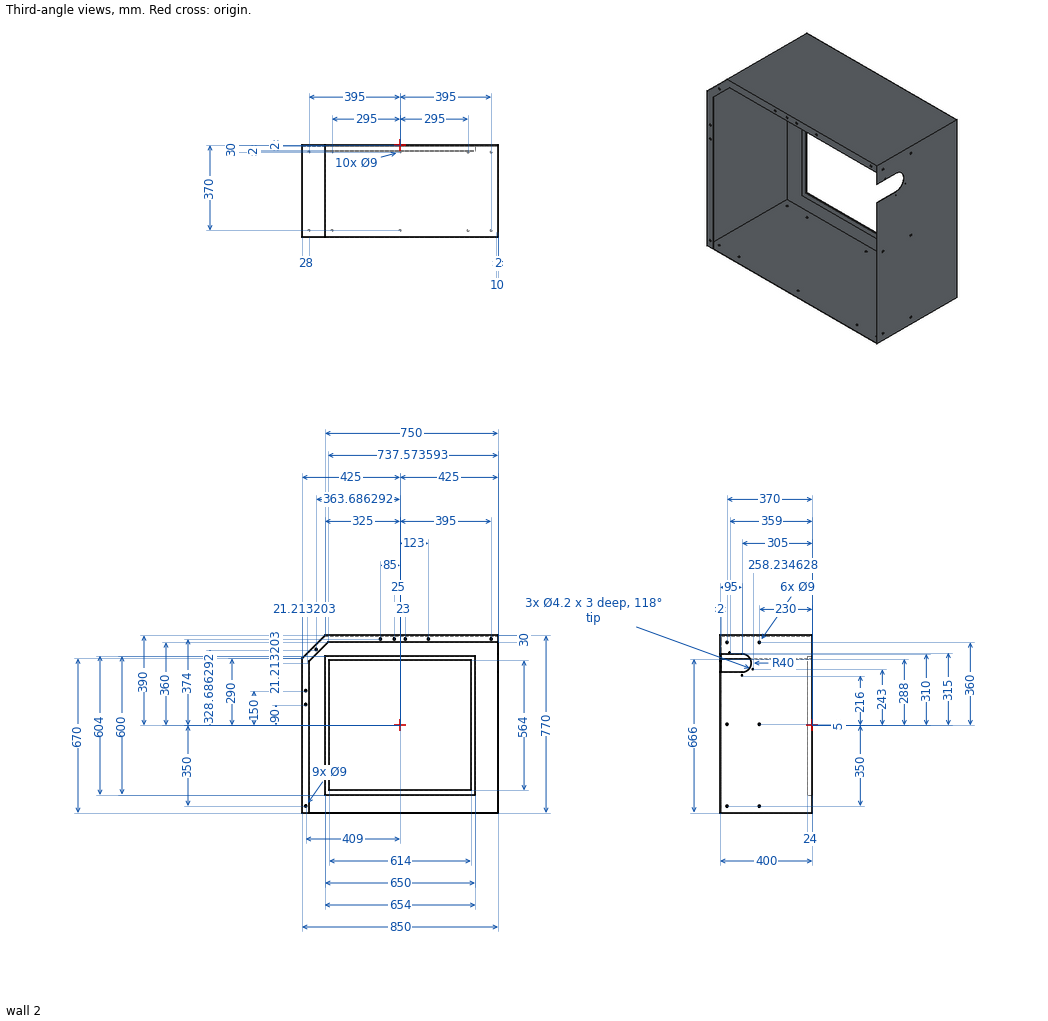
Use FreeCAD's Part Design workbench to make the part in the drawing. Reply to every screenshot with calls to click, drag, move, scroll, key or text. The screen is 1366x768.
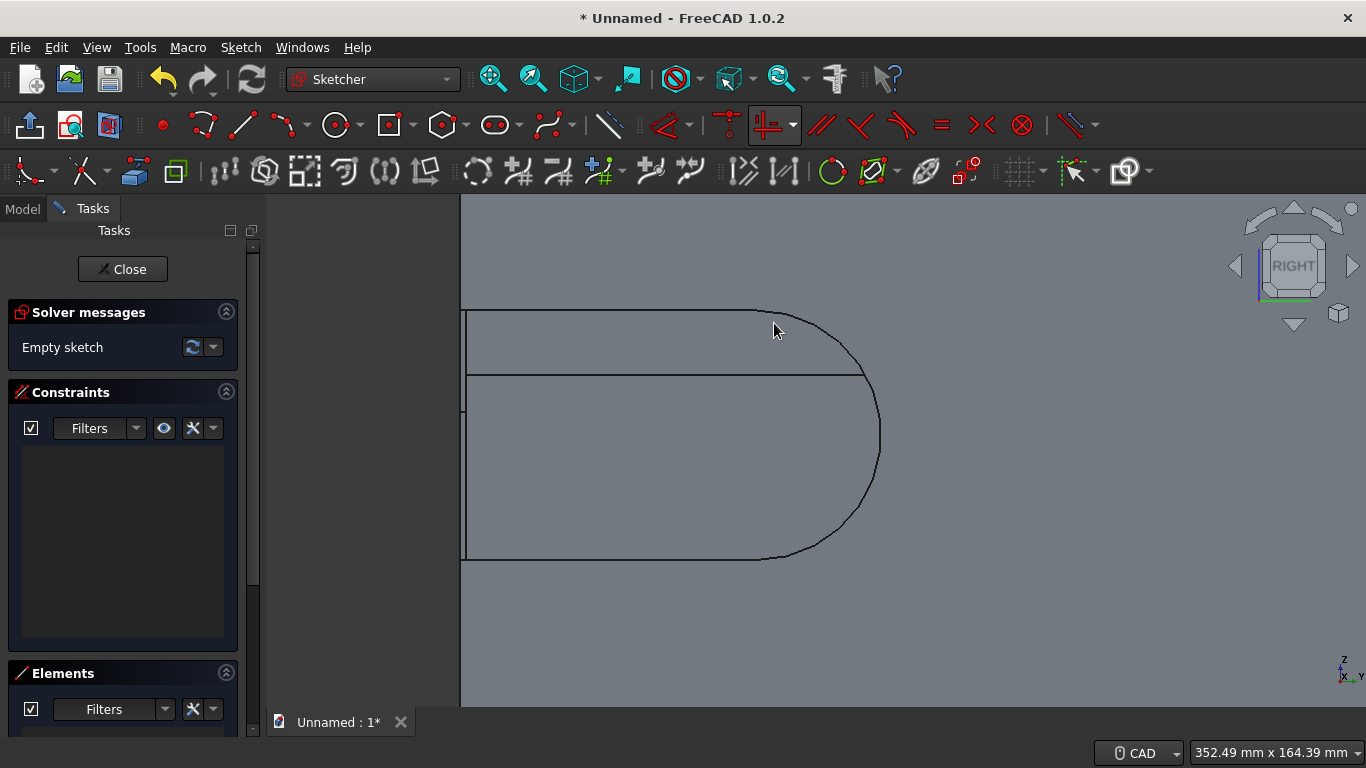
click(336, 126)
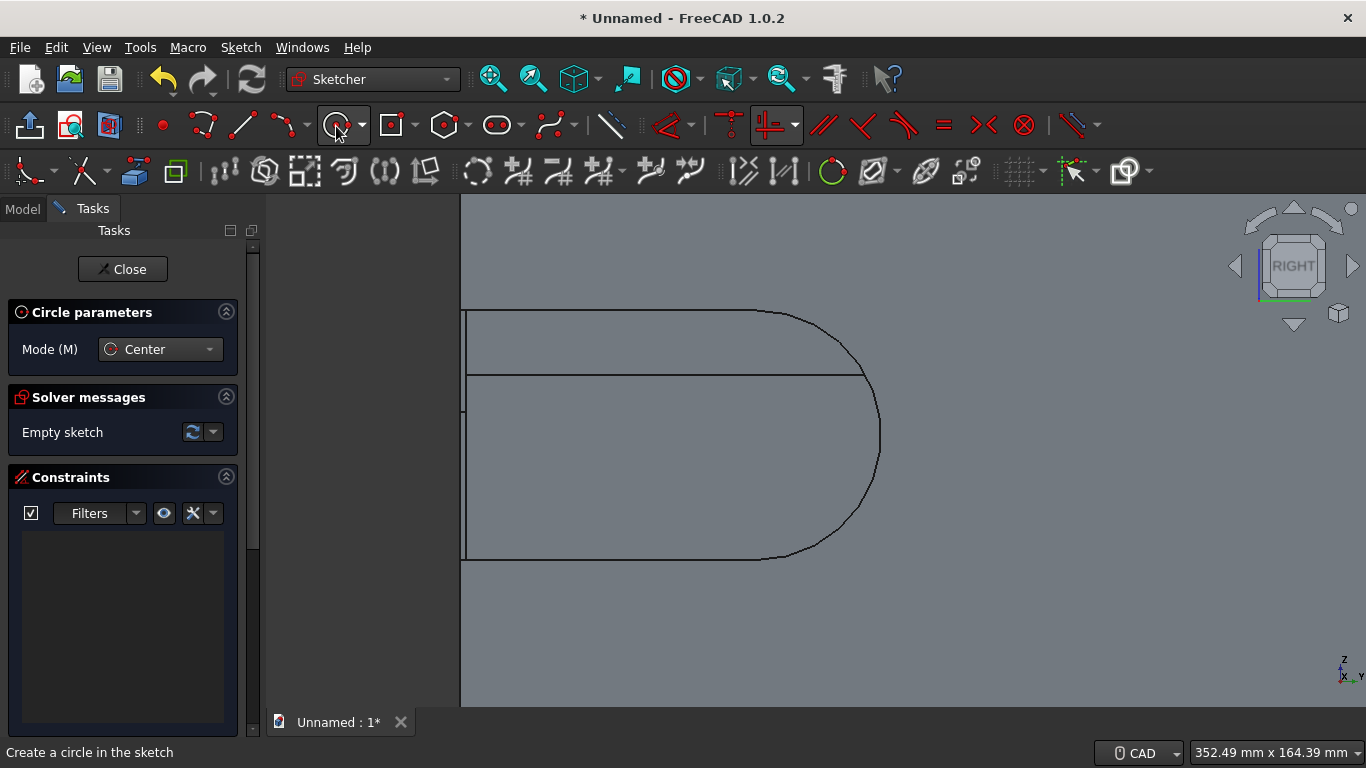
scroll(902, 520, up, 7)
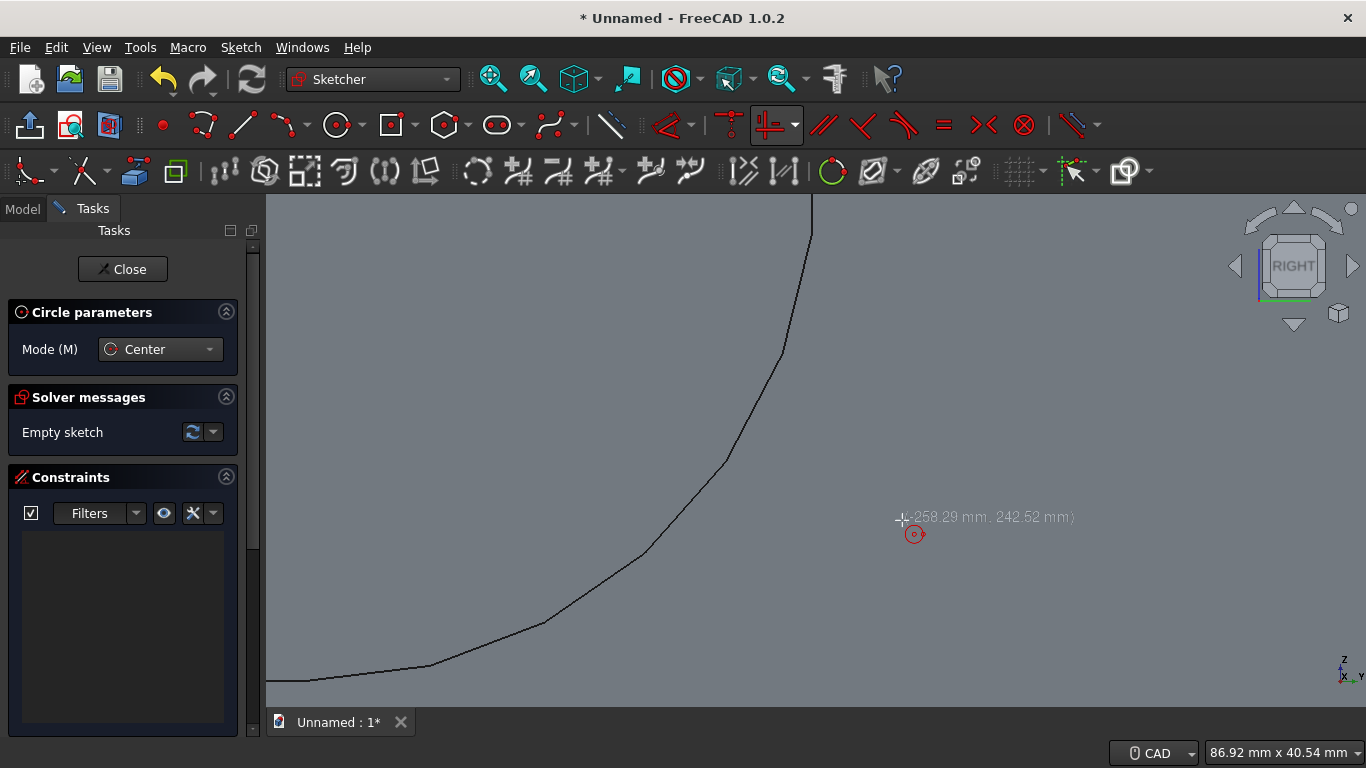
scroll(906, 522, down, 7)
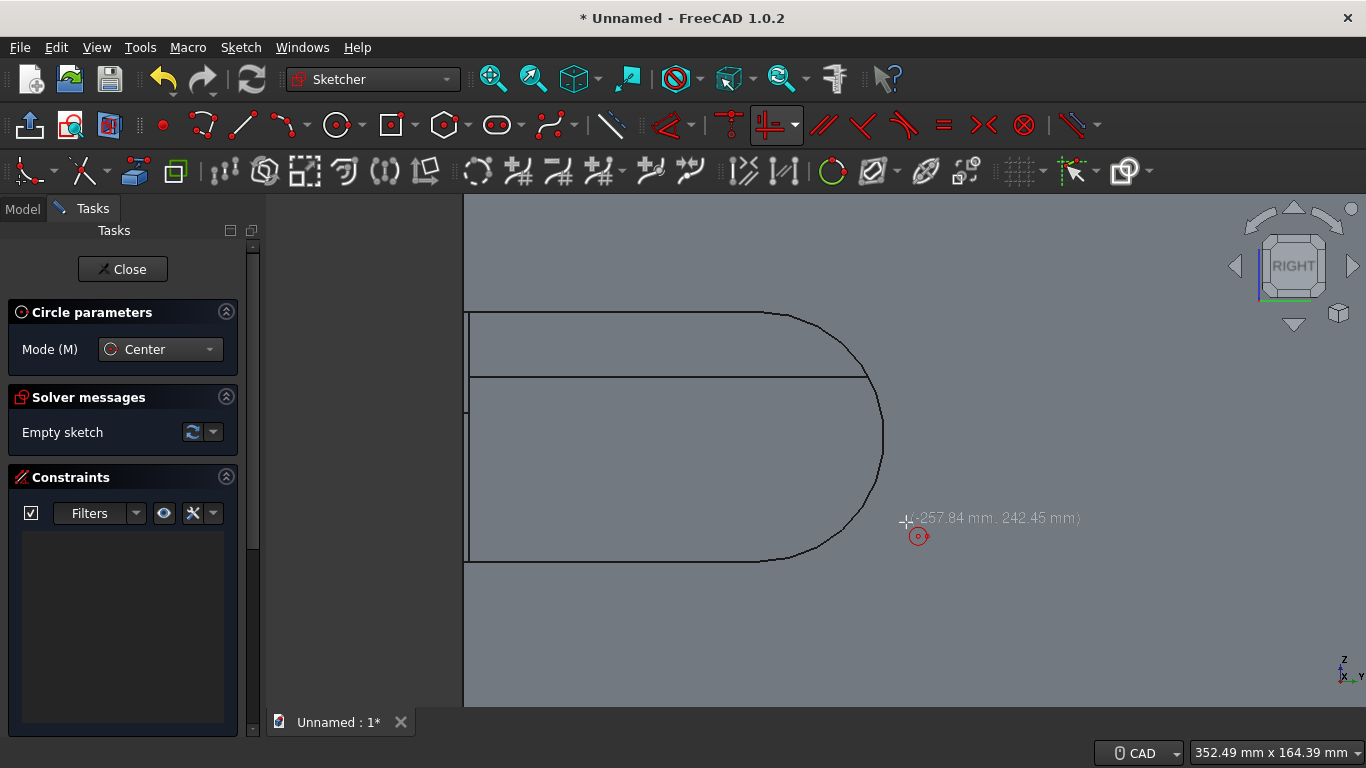
click(905, 521)
move(910, 516)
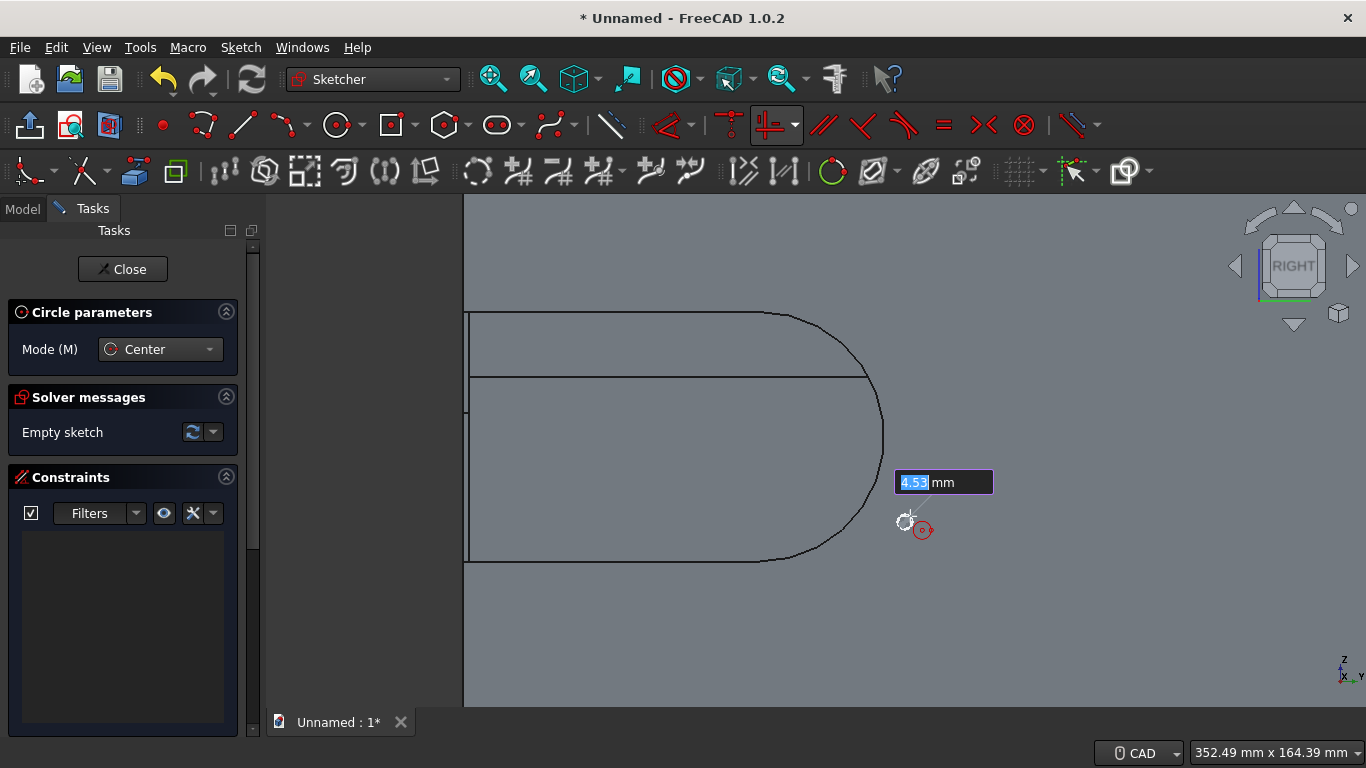
text(4.2)
key(Return)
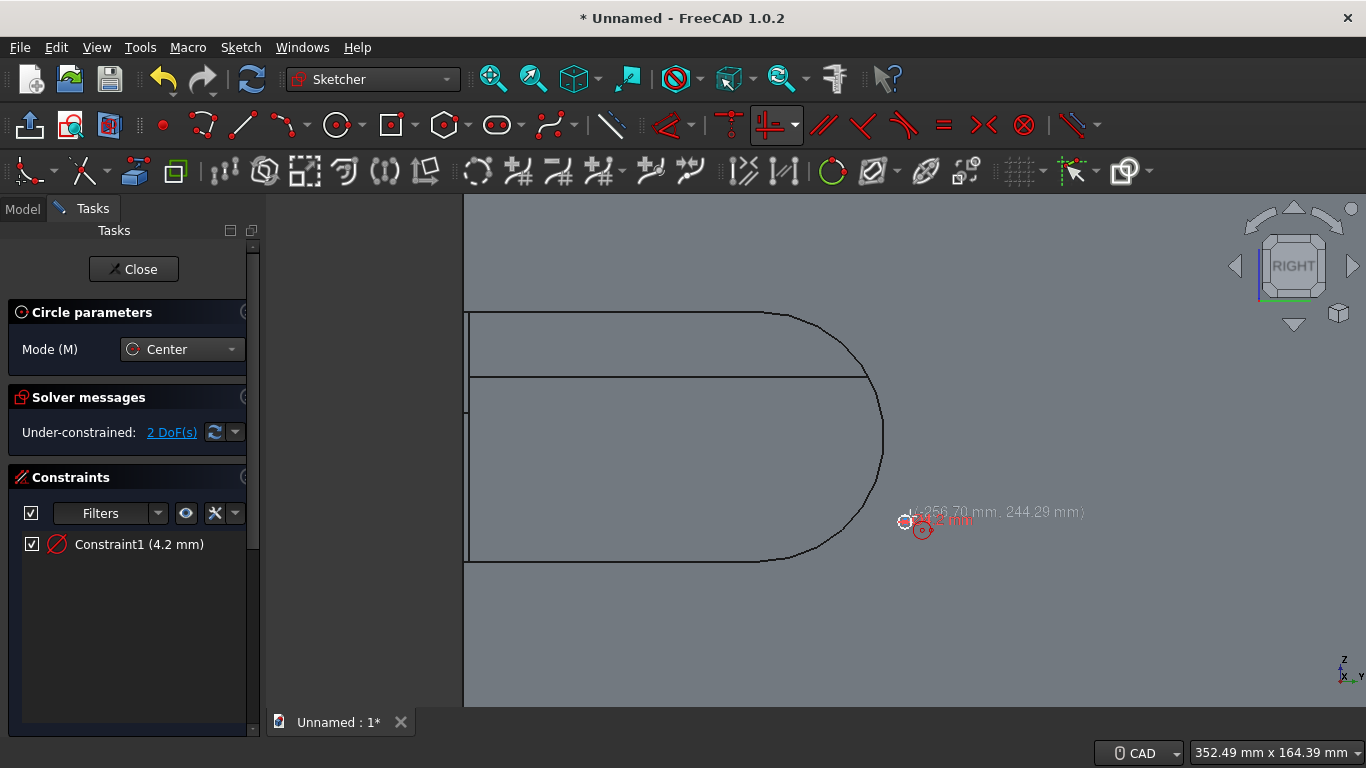
scroll(759, 605, up, 7)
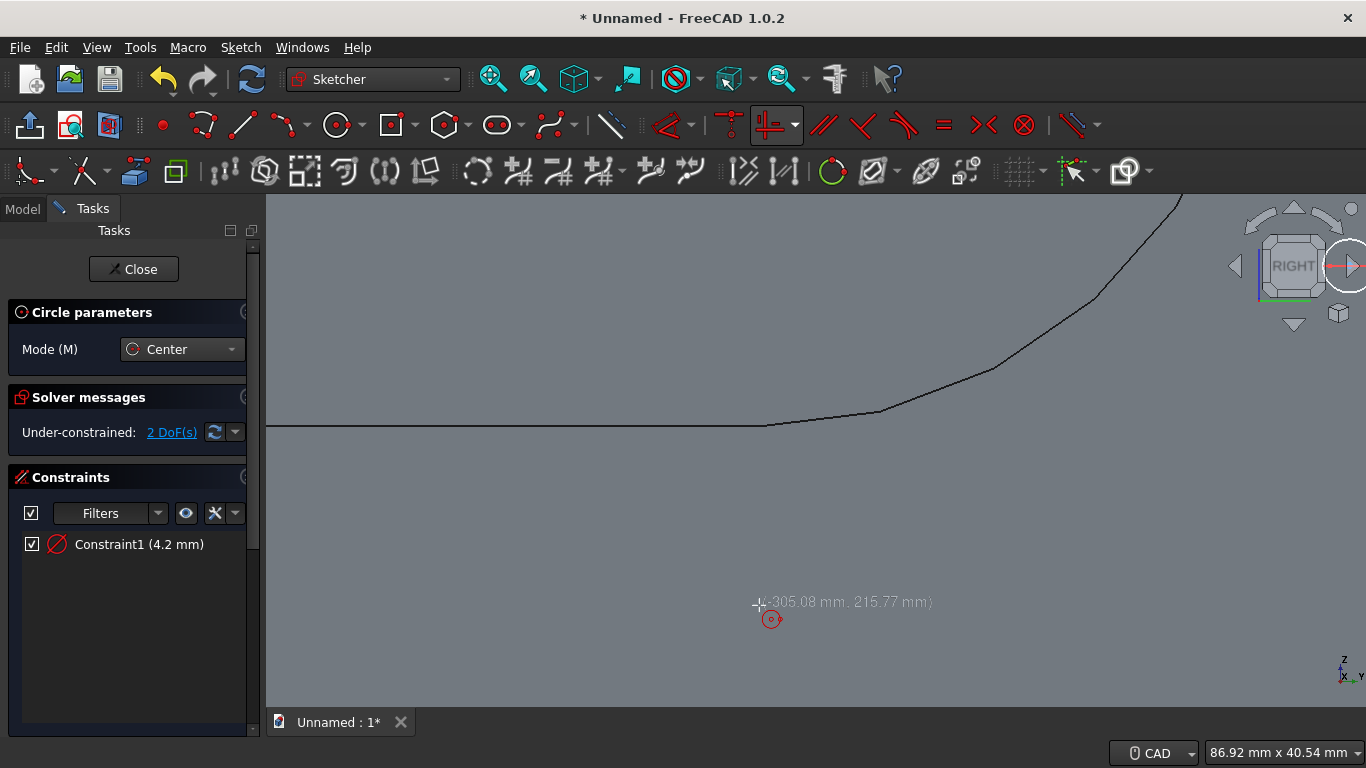
scroll(759, 605, down, 7)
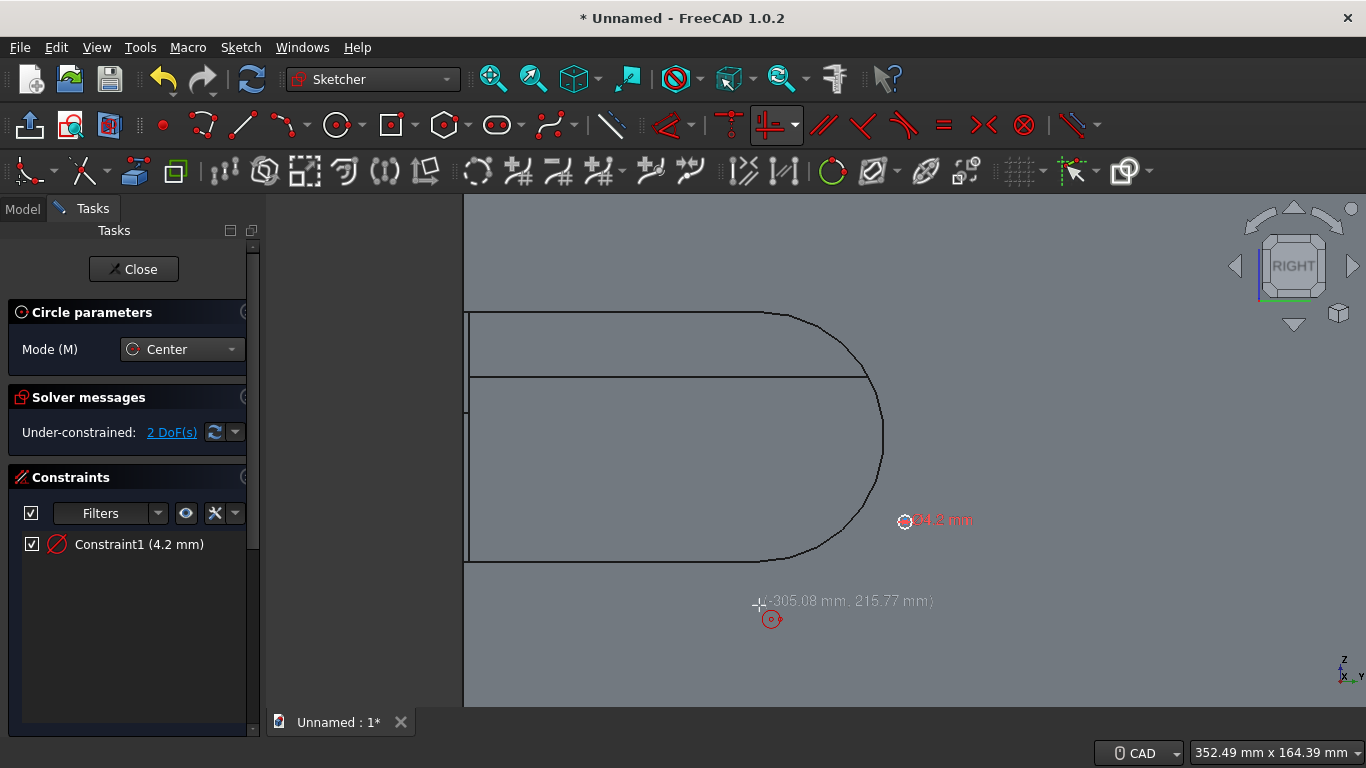
click(759, 605)
move(764, 601)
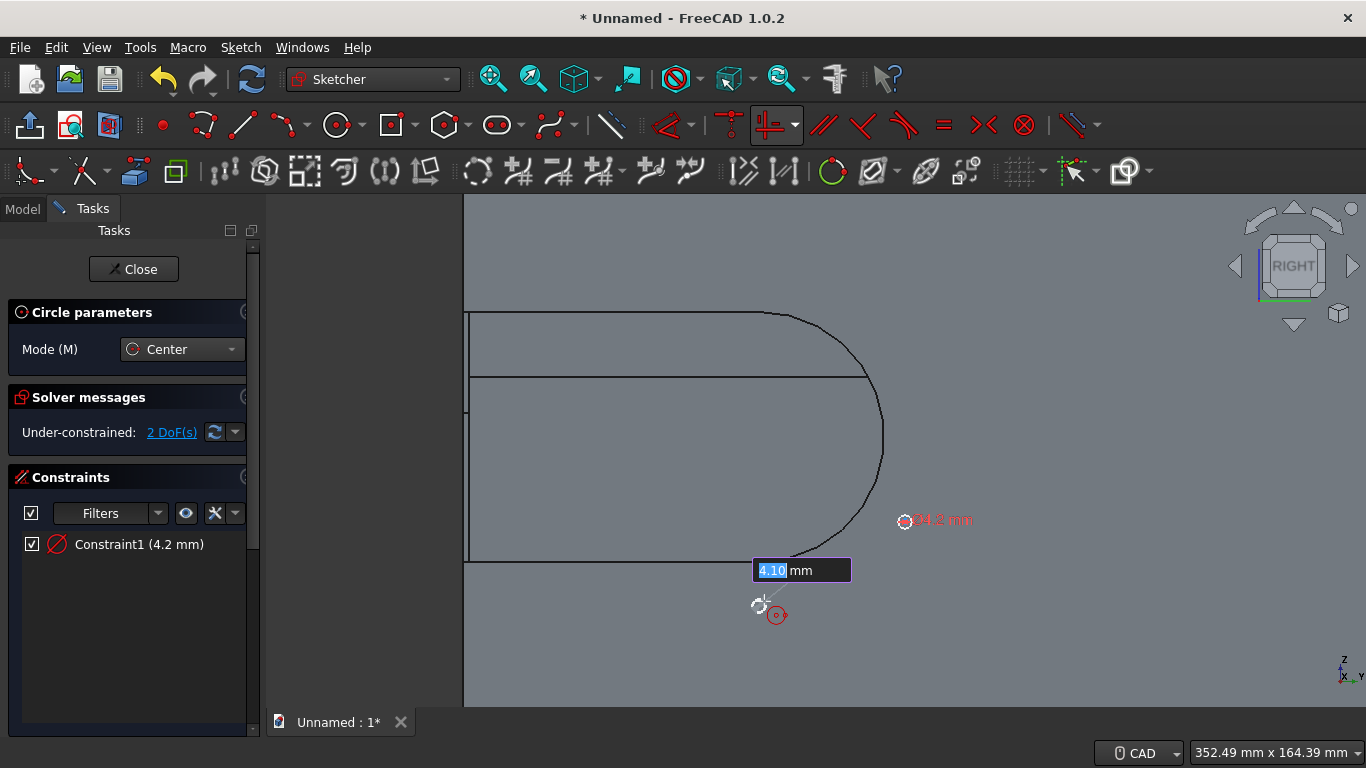
text(4.2)
key(Return)